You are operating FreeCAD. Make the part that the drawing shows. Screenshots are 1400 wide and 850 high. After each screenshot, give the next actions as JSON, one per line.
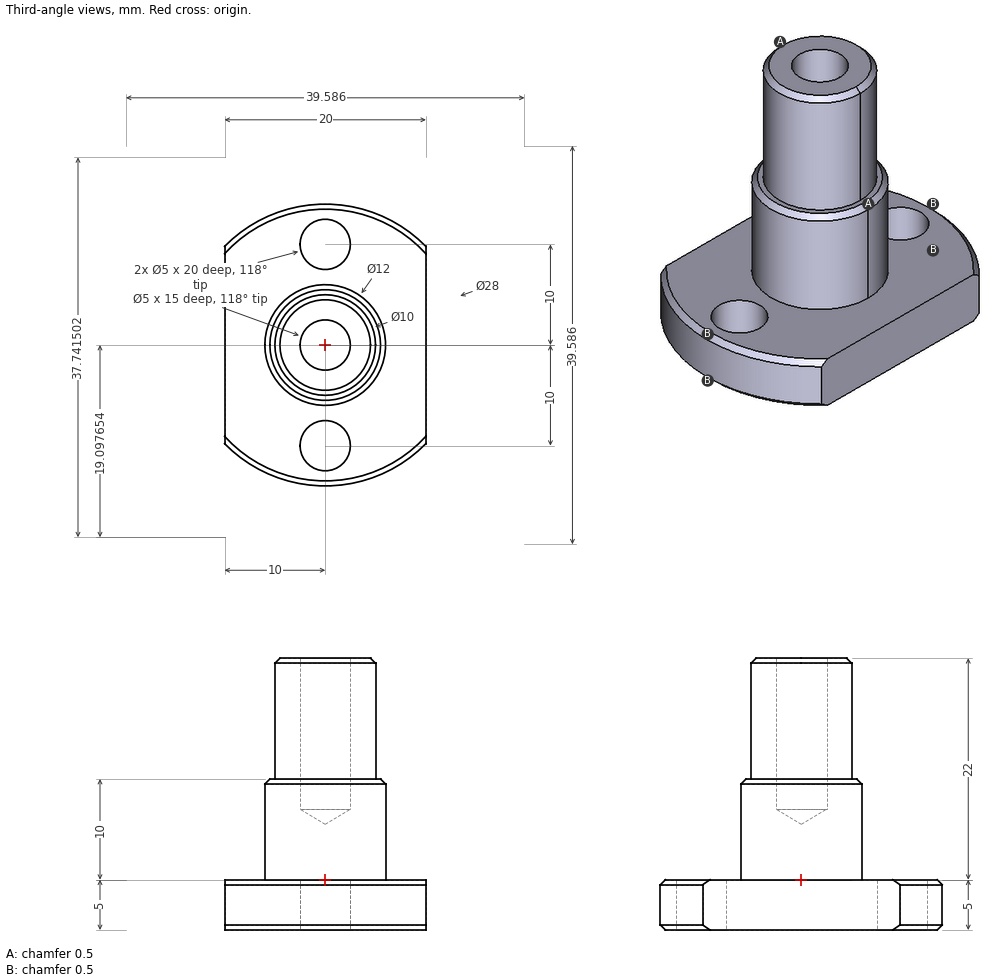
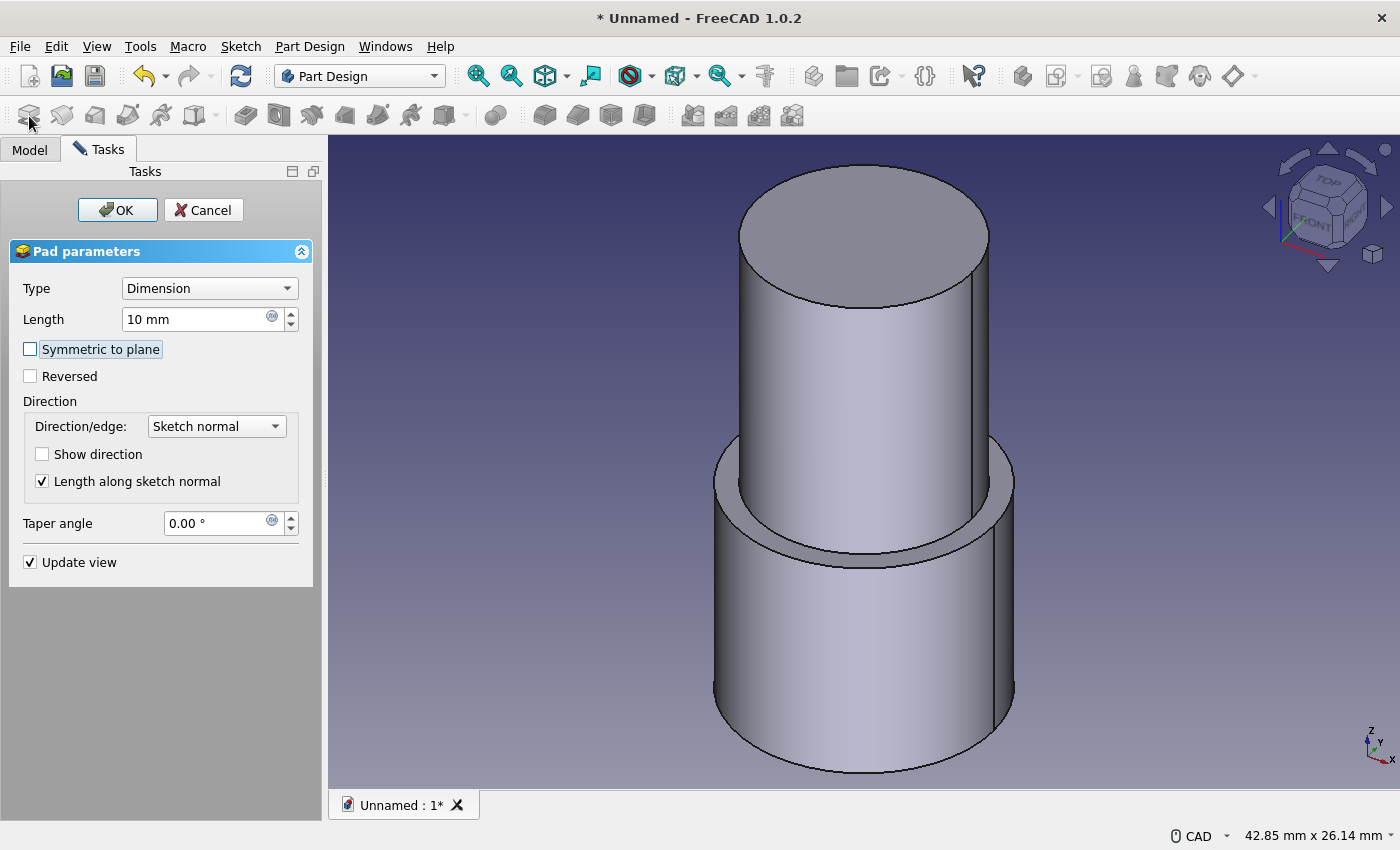
{"action": "left_click", "coordinate": [118, 210]}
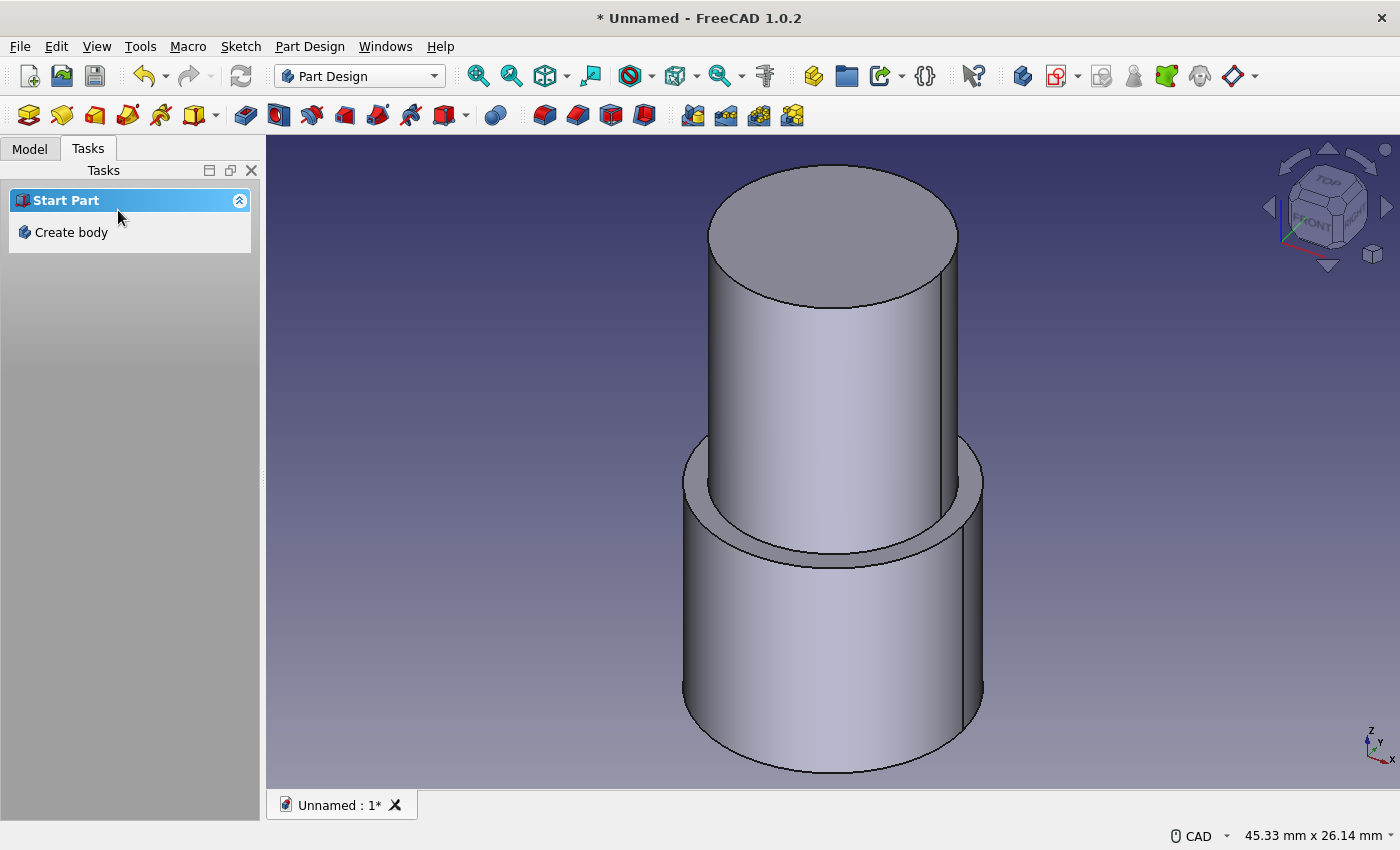
{"action": "left_click", "coordinate": [479, 76]}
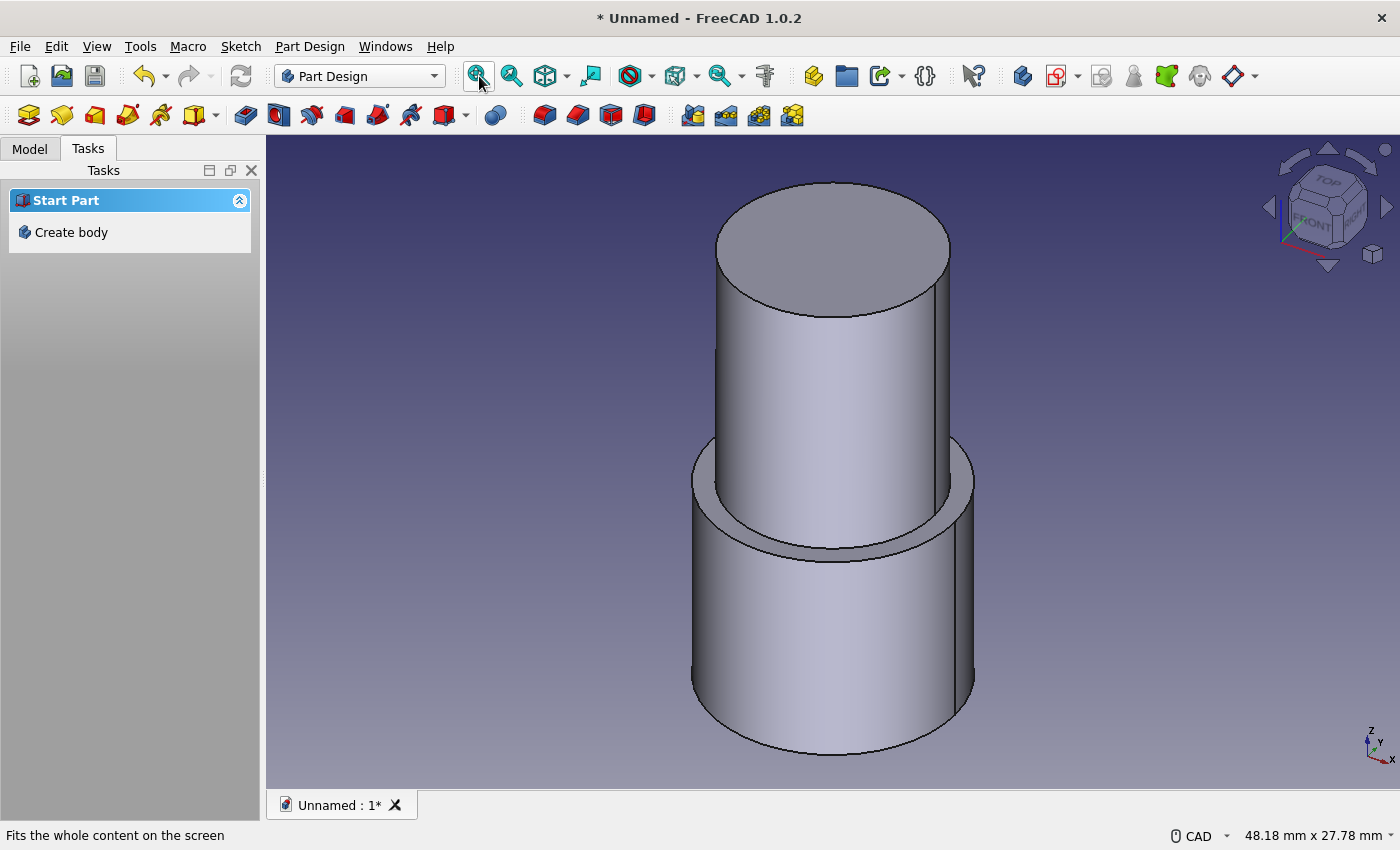
{"action": "left_click", "coordinate": [1056, 76]}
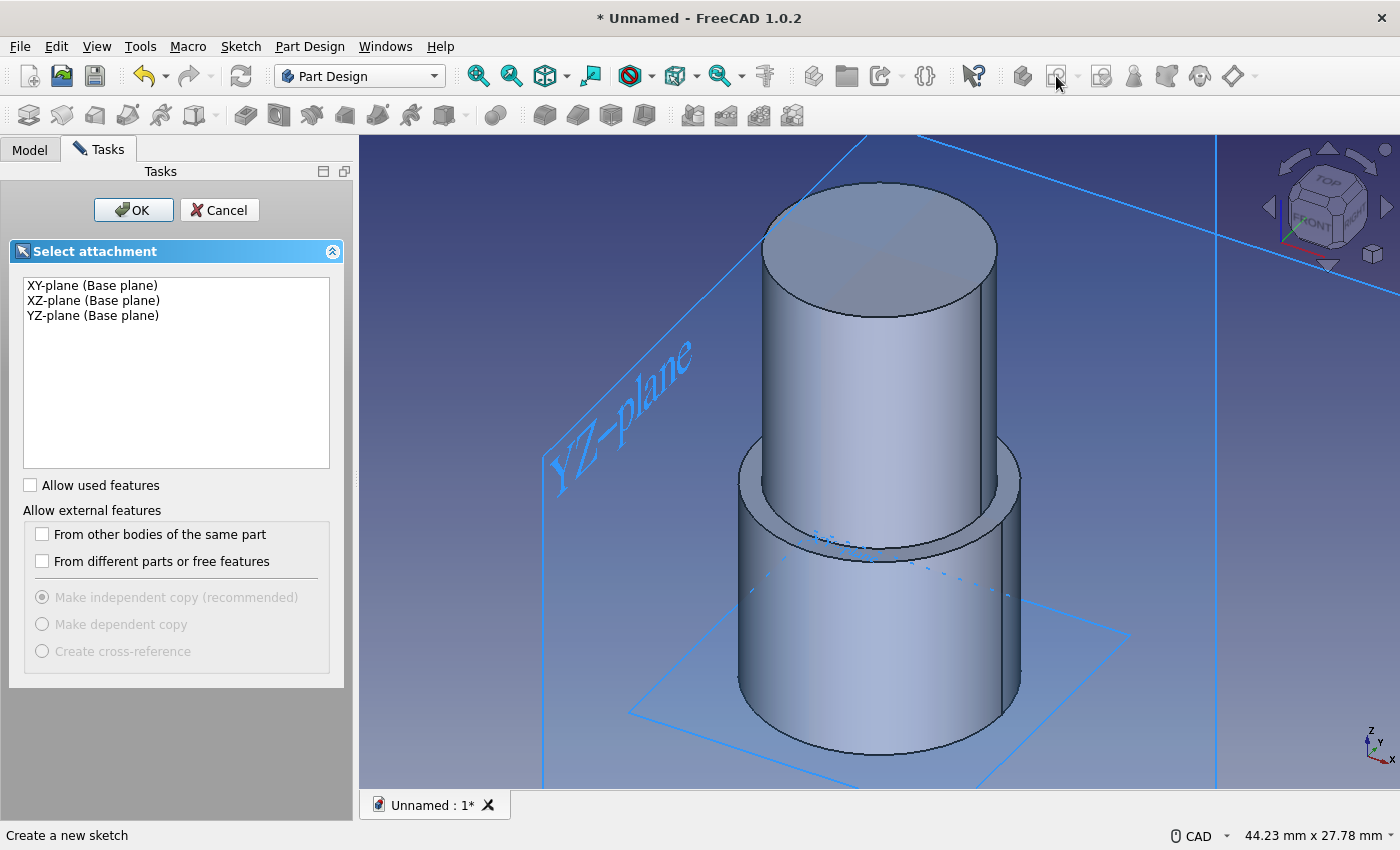
{"action": "left_click", "coordinate": [84, 286]}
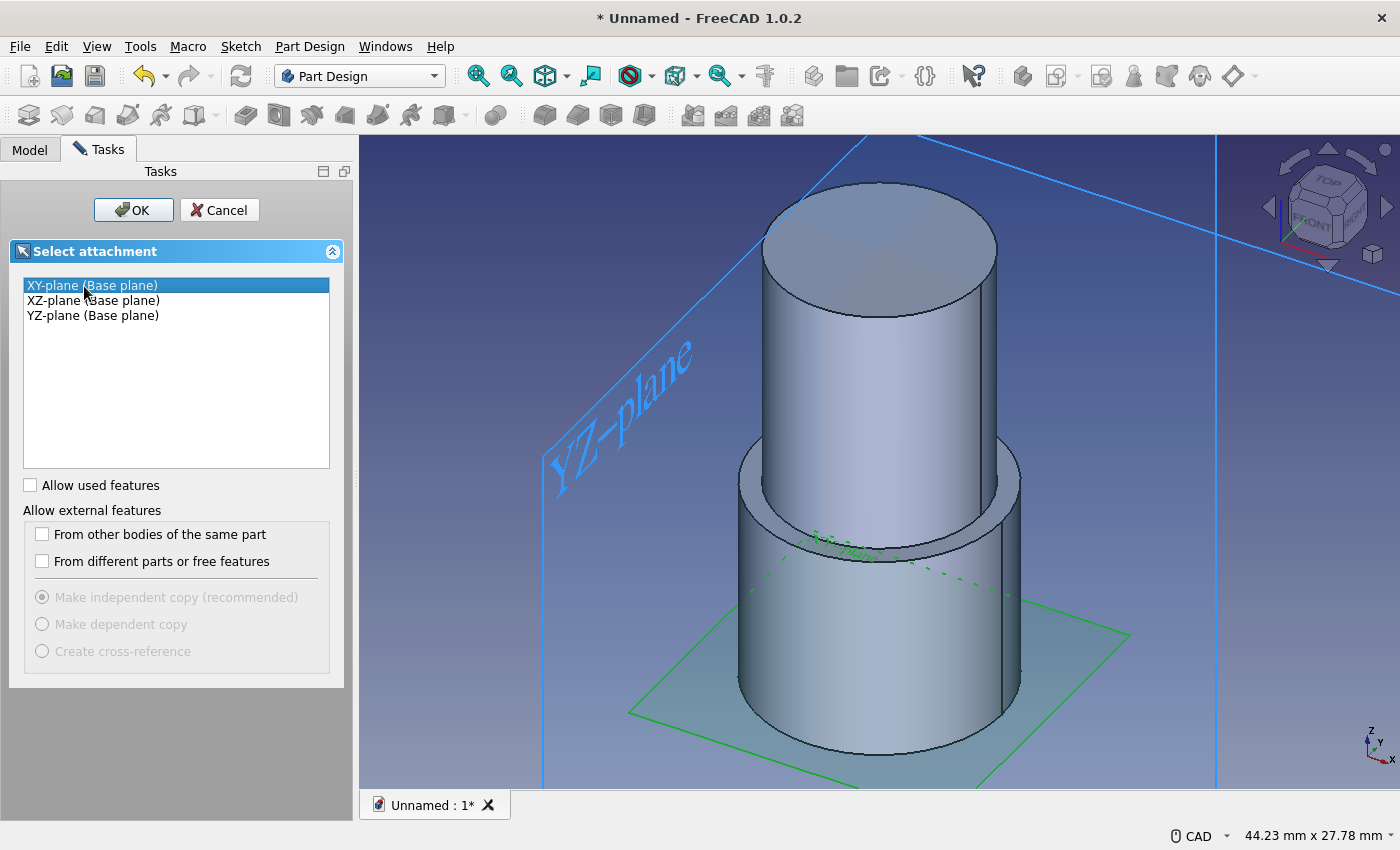
{"action": "left_click", "coordinate": [134, 210]}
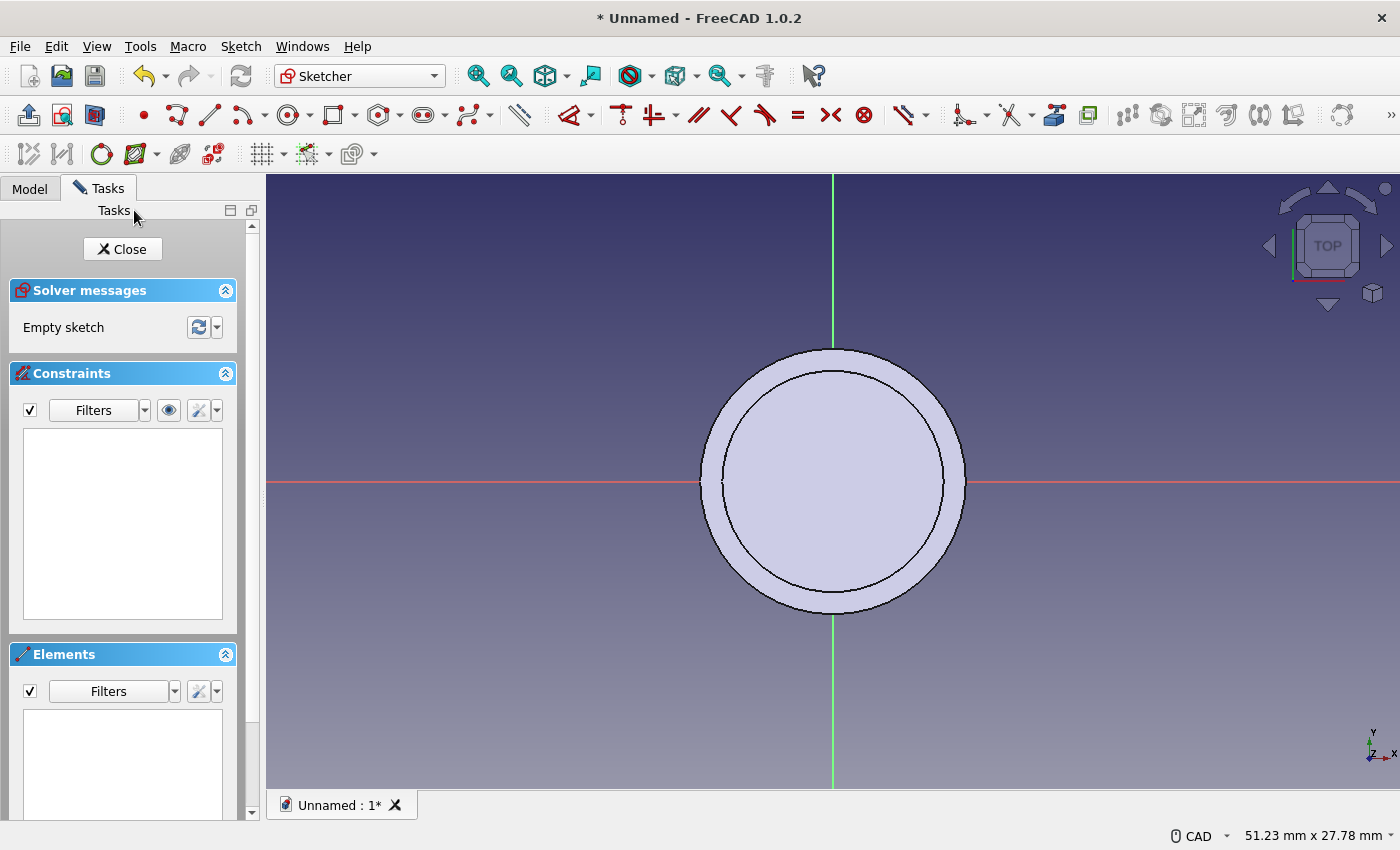
{"action": "key", "text": "q s"}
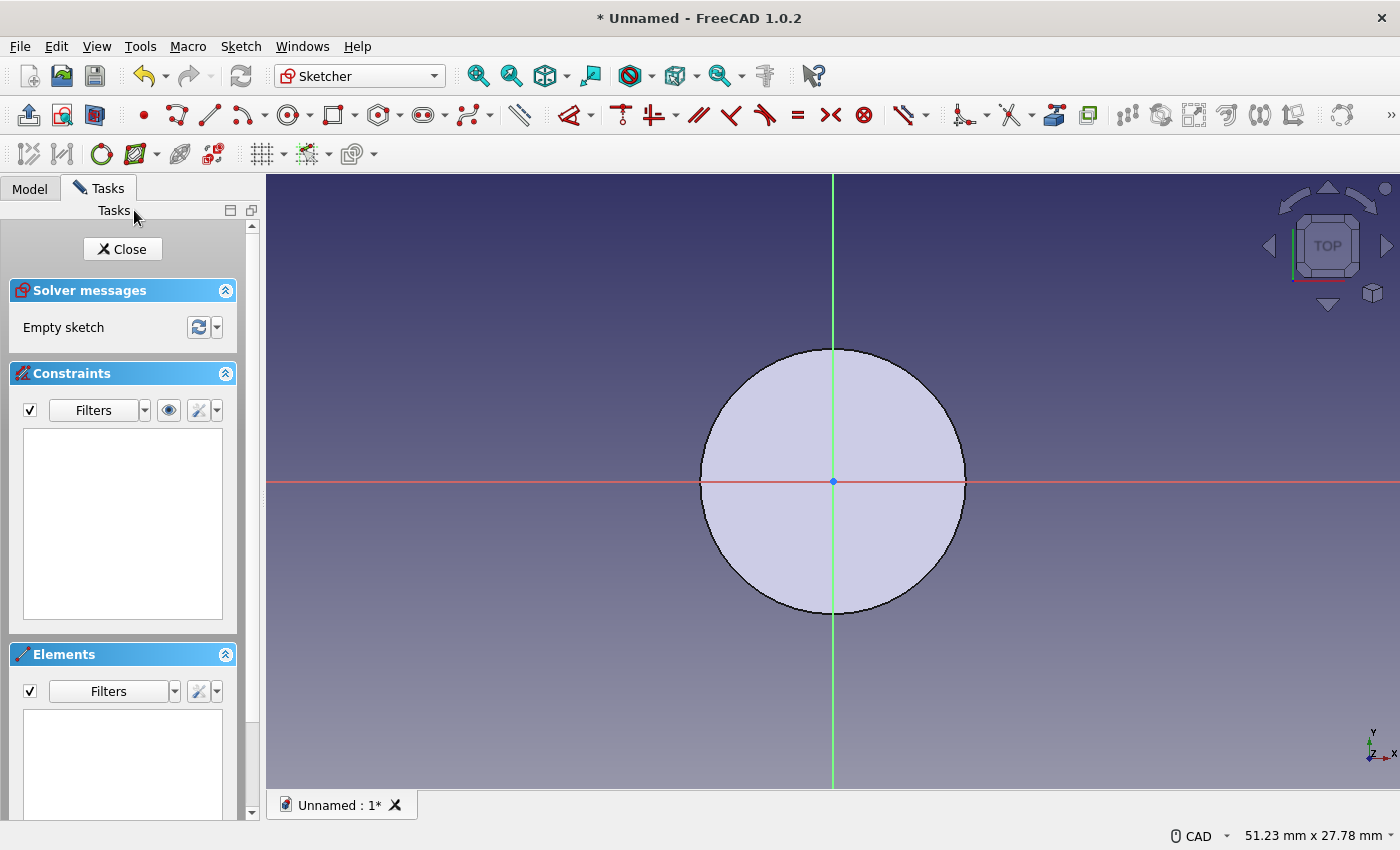
{"action": "scroll", "coordinate": [625, 481], "scroll_direction": "down", "scroll_amount": 2}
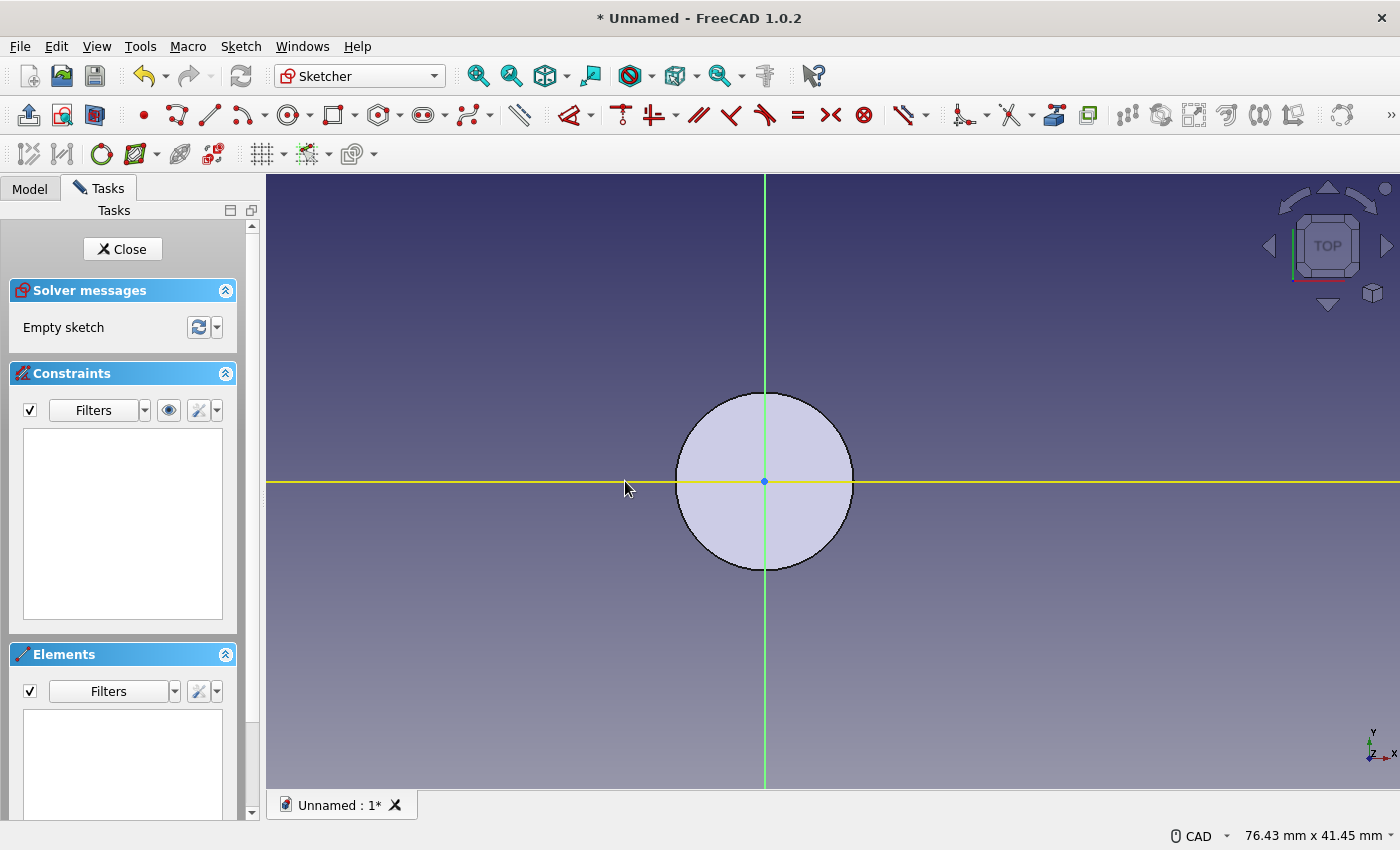
{"action": "key", "text": "g c"}